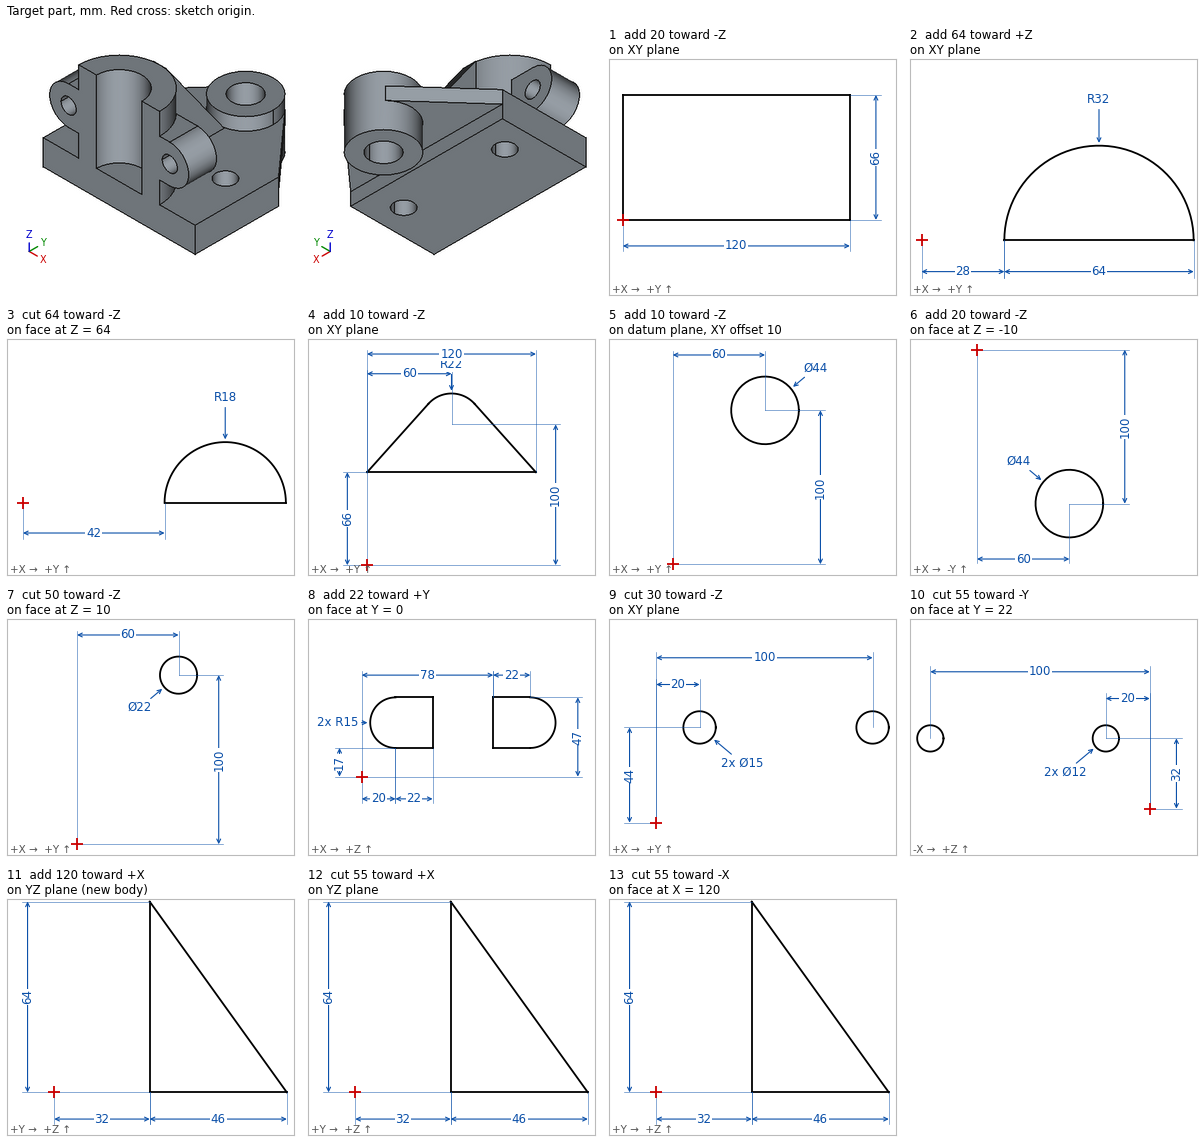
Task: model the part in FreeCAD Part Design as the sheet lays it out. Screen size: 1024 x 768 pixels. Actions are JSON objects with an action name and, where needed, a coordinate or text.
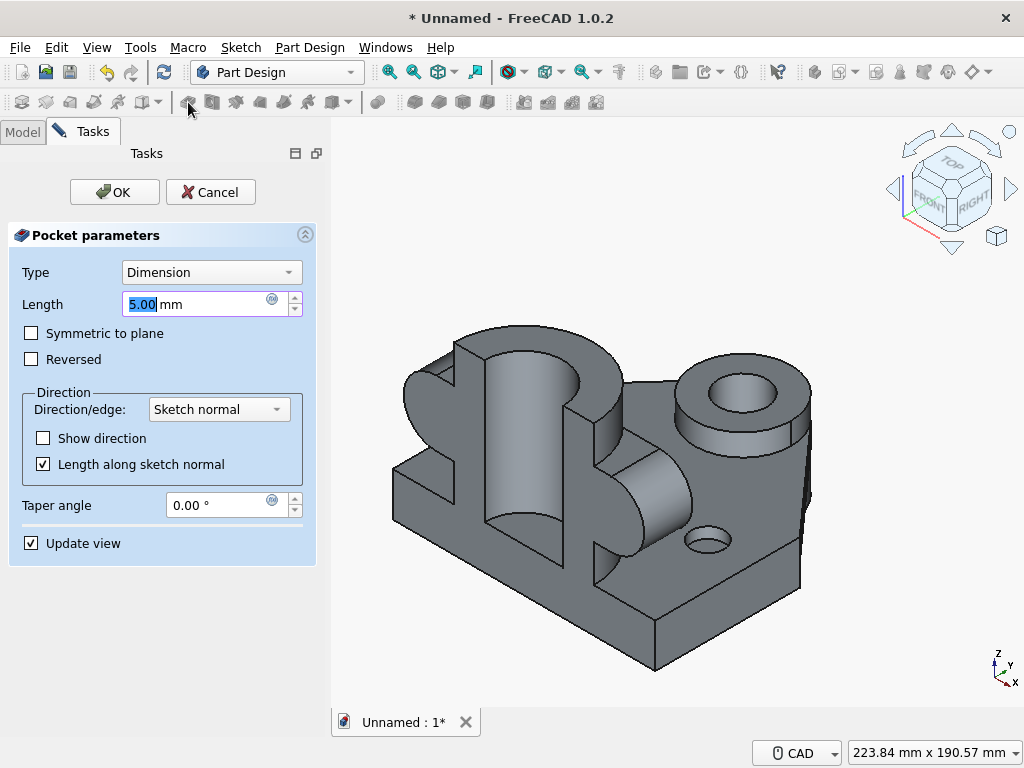
{"action": "type", "text": "30"}
{"action": "key", "text": "Tab"}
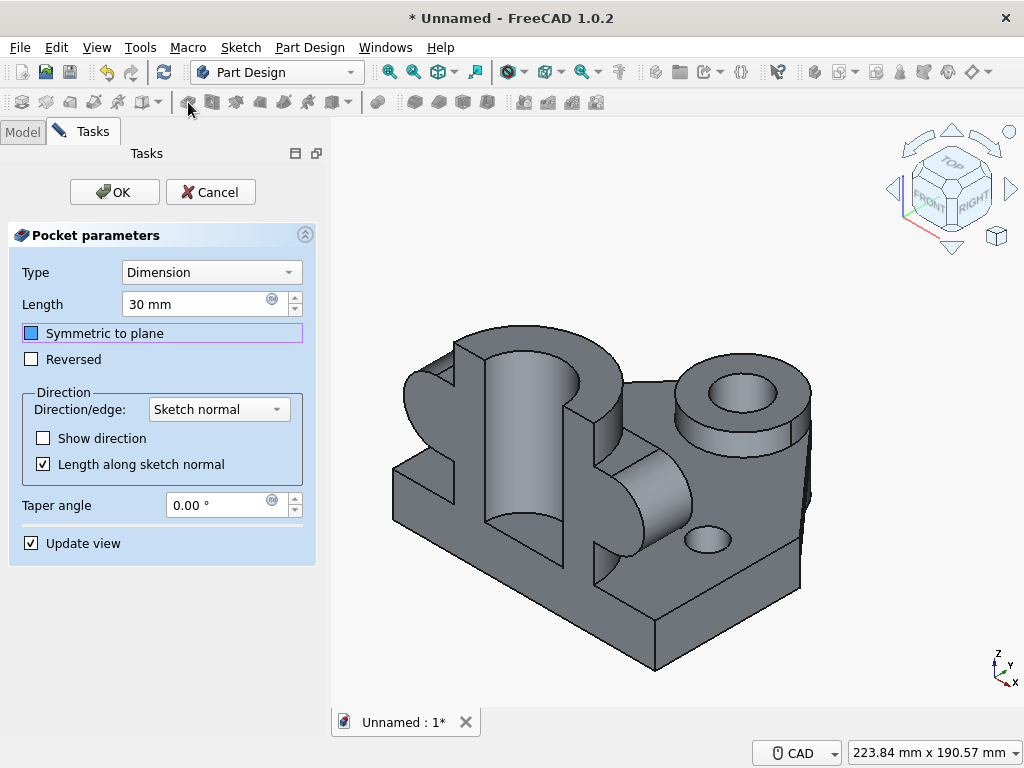
{"action": "left_click", "coordinate": [115, 192]}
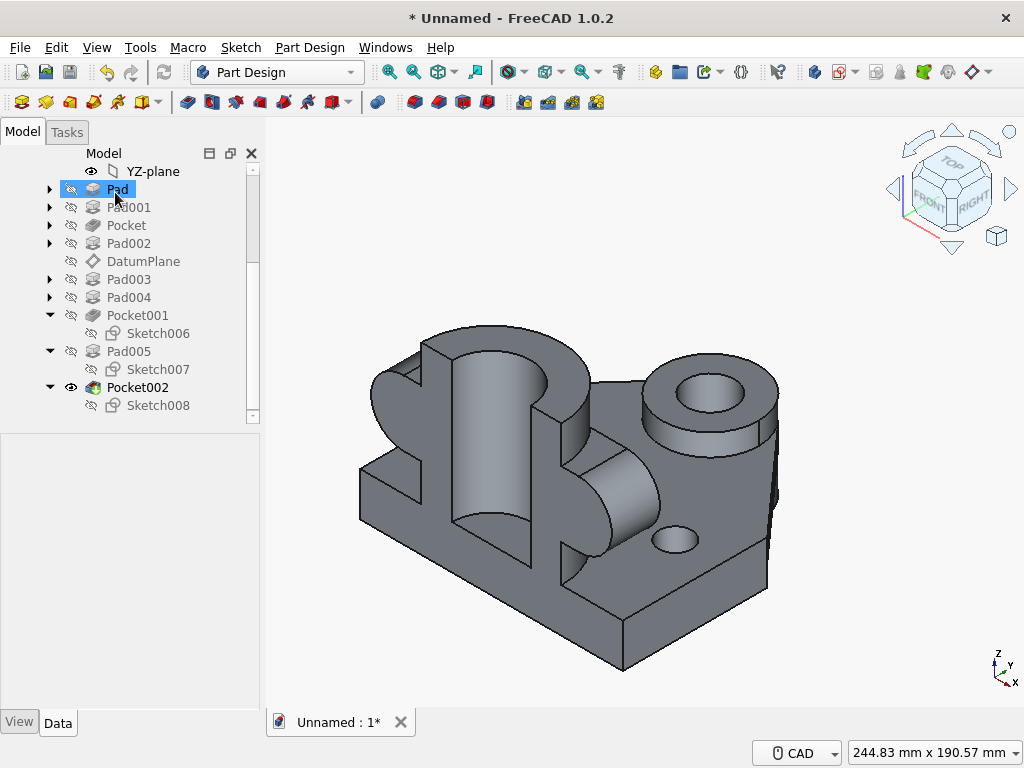
{"action": "key", "text": "4"}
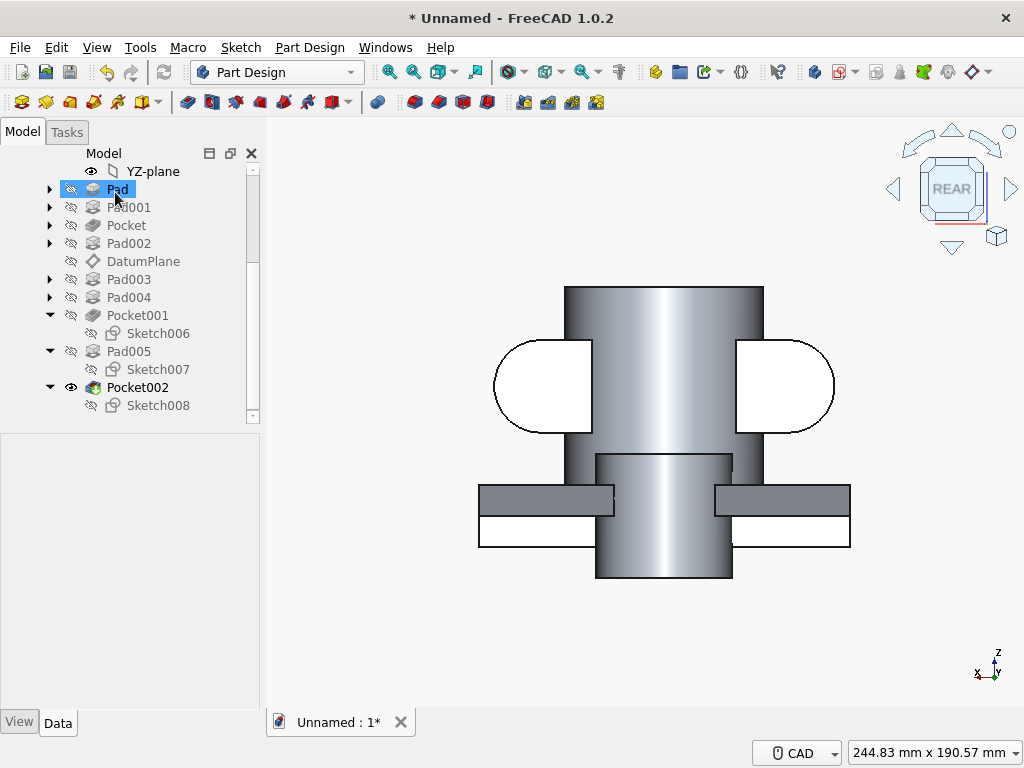
{"action": "left_click", "coordinate": [543, 385]}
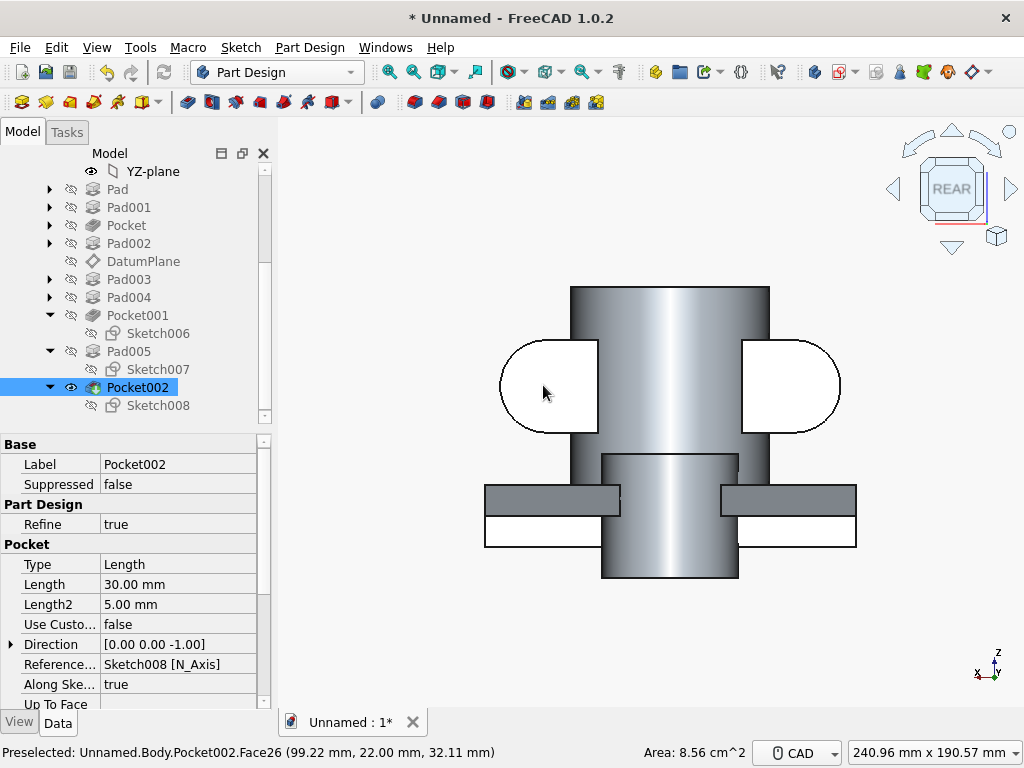
{"action": "left_click", "coordinate": [840, 72]}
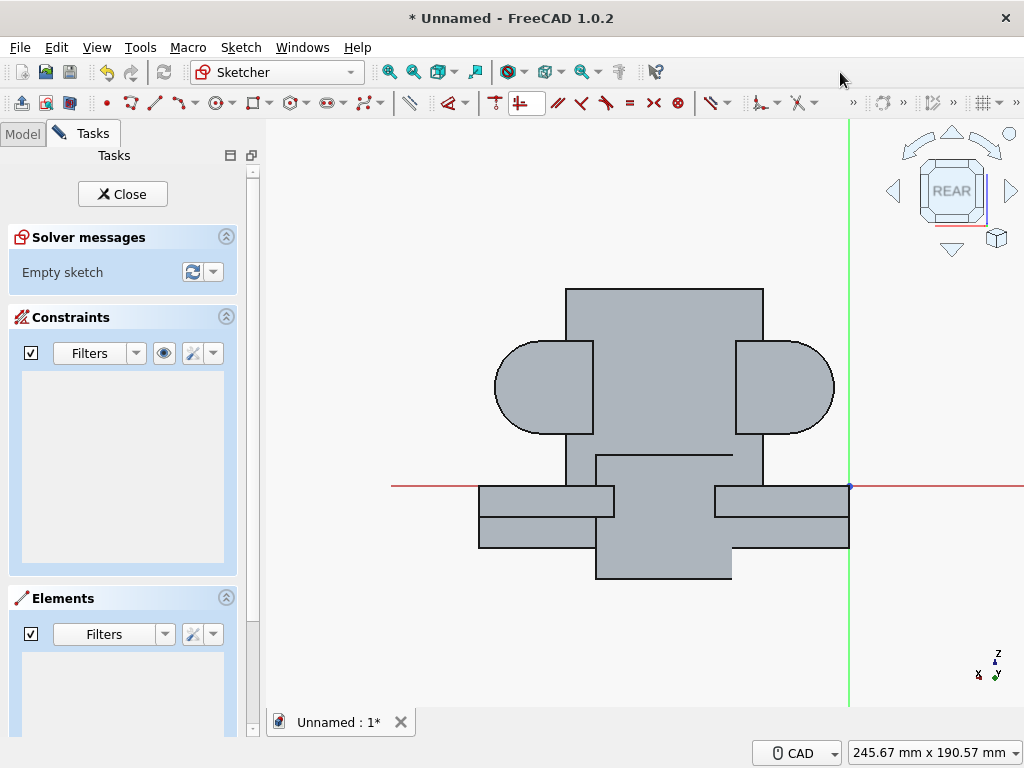
{"action": "left_click", "coordinate": [70, 104]}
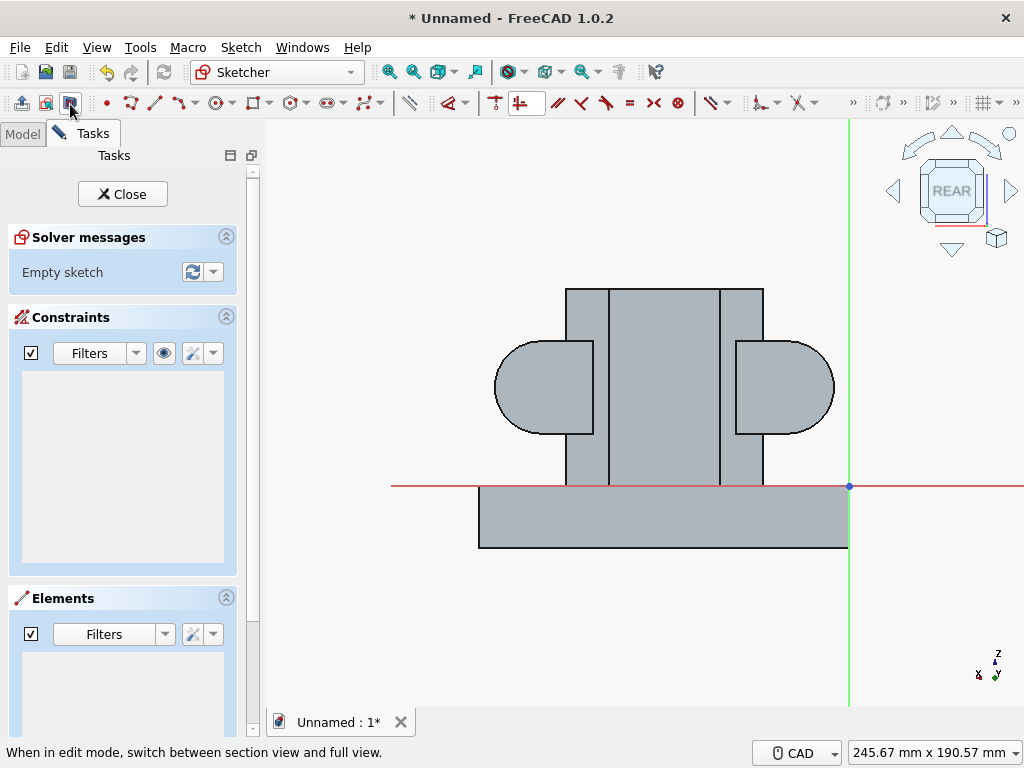
{"action": "scroll", "coordinate": [294, 347], "scroll_direction": "down", "scroll_amount": 1}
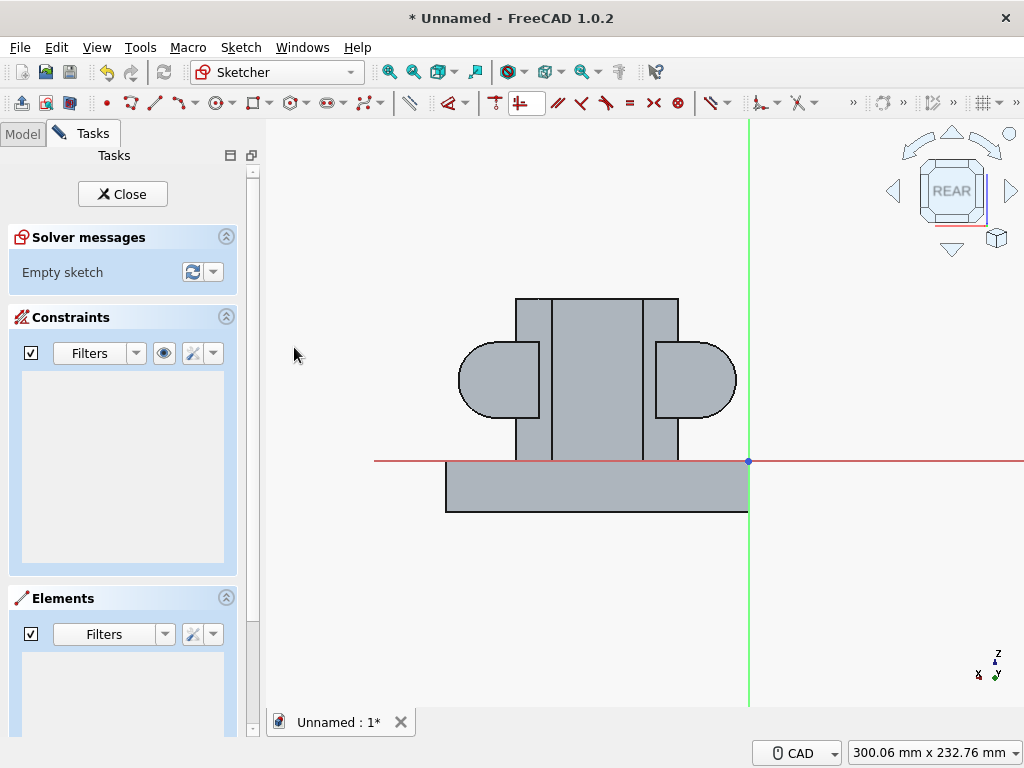
{"action": "scroll", "coordinate": [693, 413], "scroll_direction": "up", "scroll_amount": 2}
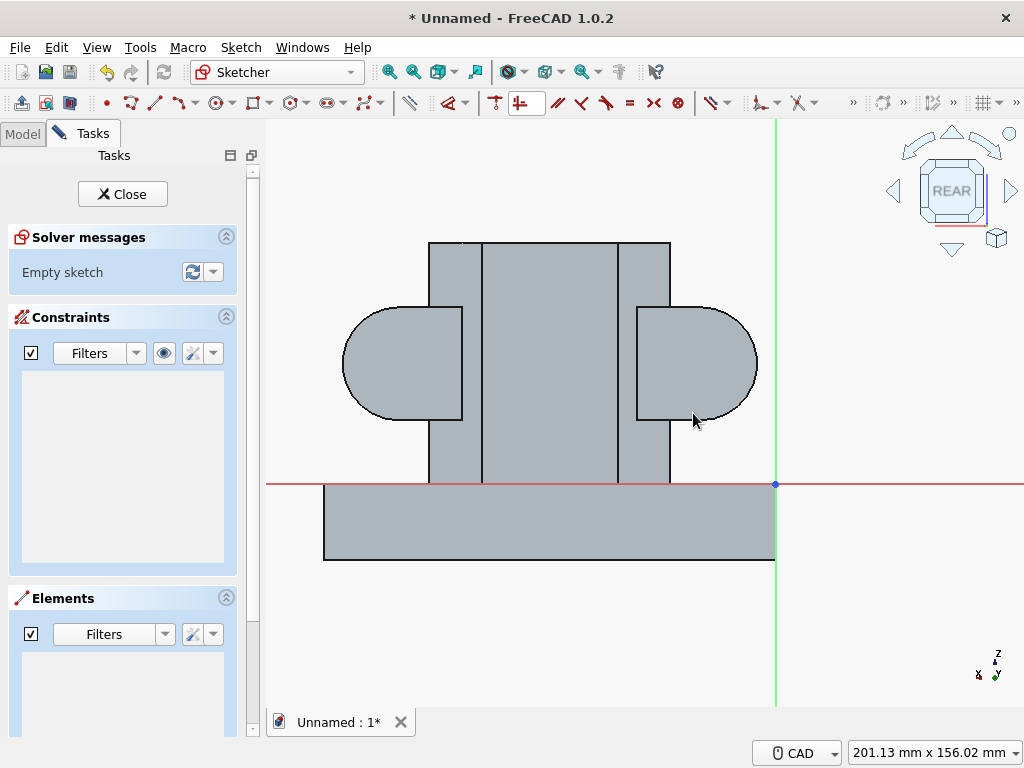
{"action": "left_click", "coordinate": [216, 104]}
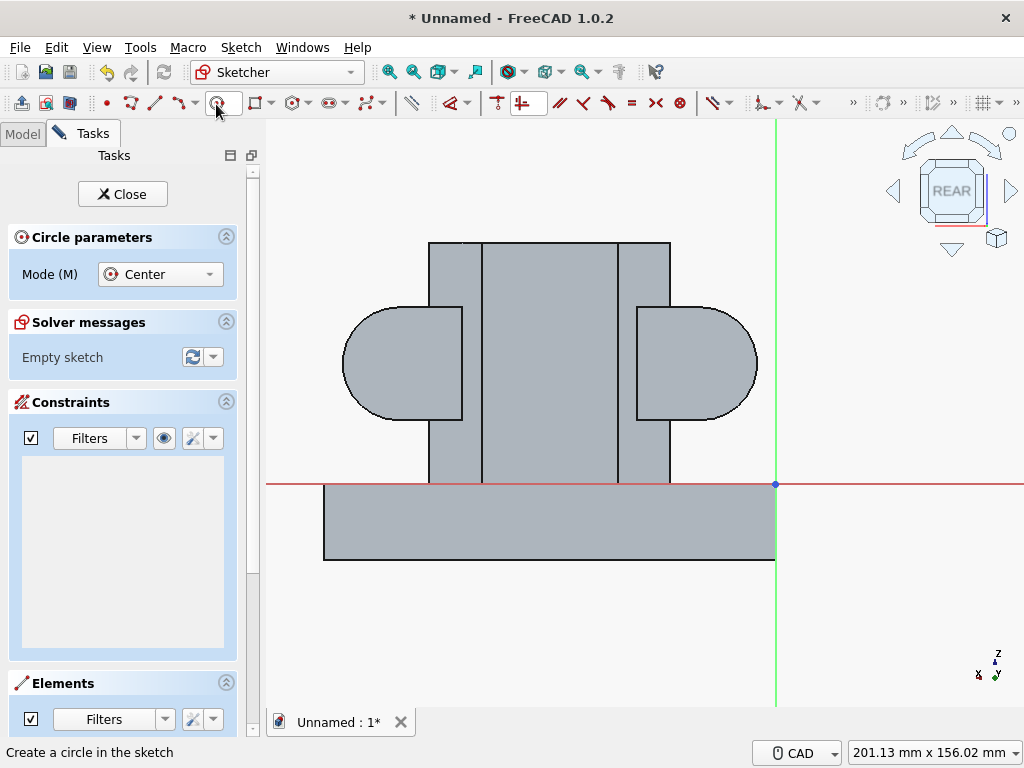
{"action": "left_click", "coordinate": [701, 364]}
{"action": "left_click", "coordinate": [717, 348]}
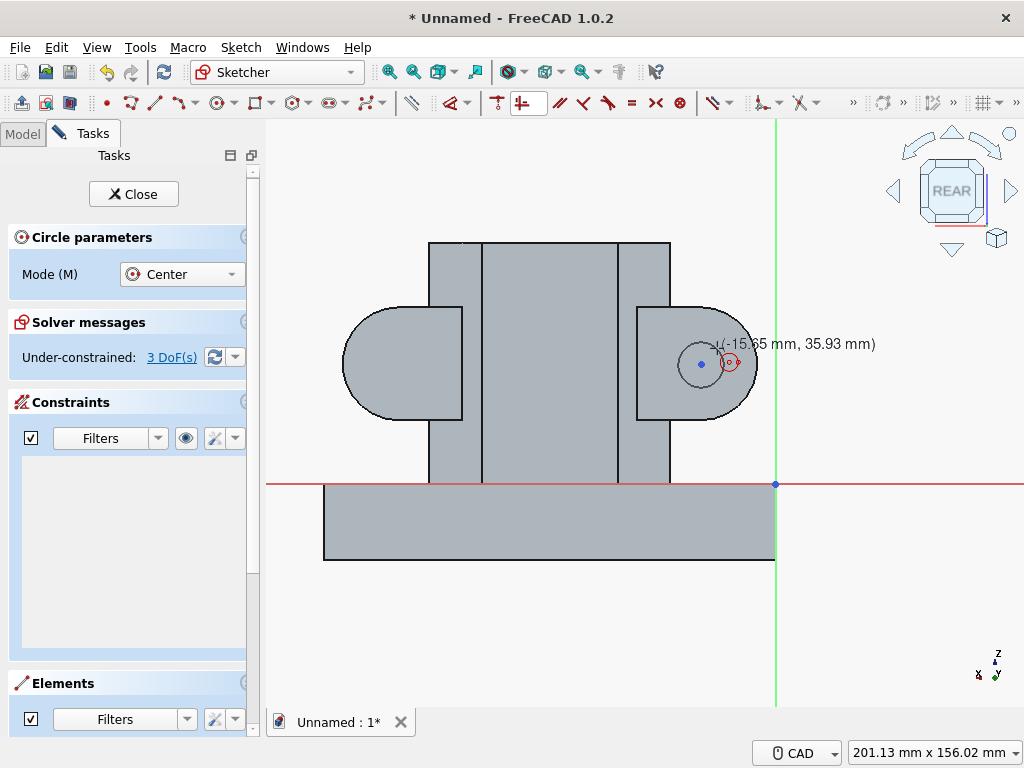
{"action": "left_click", "coordinate": [399, 364]}
{"action": "left_click", "coordinate": [415, 348]}
{"action": "key", "text": "Escape"}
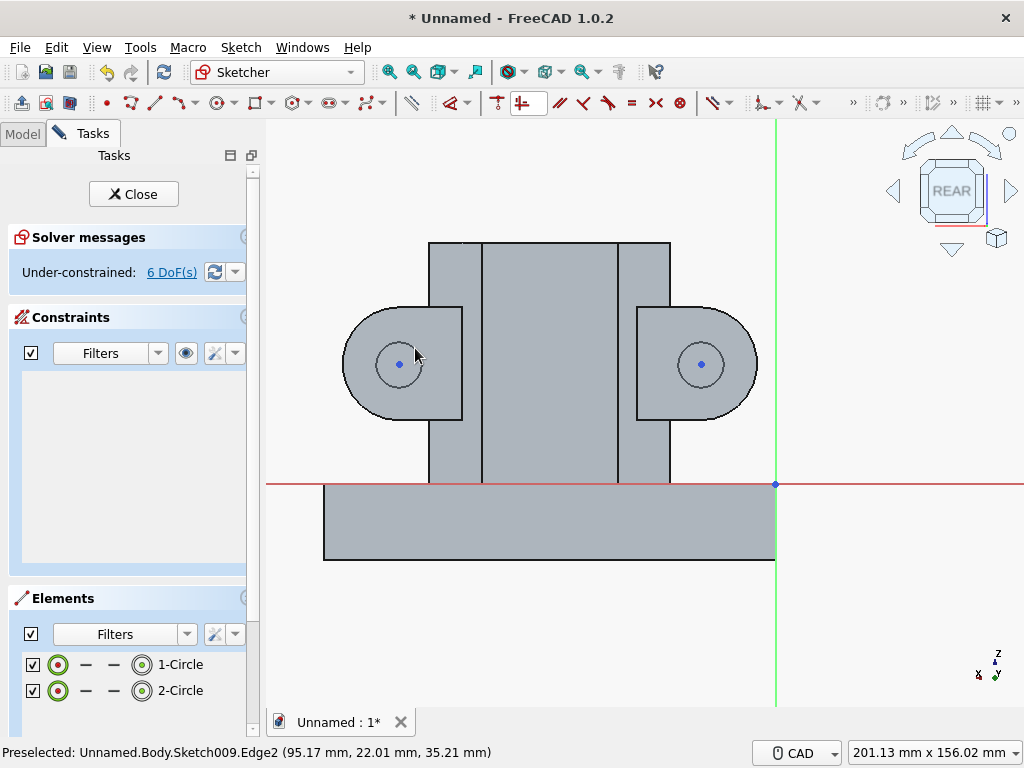
{"action": "left_click", "coordinate": [717, 349]}